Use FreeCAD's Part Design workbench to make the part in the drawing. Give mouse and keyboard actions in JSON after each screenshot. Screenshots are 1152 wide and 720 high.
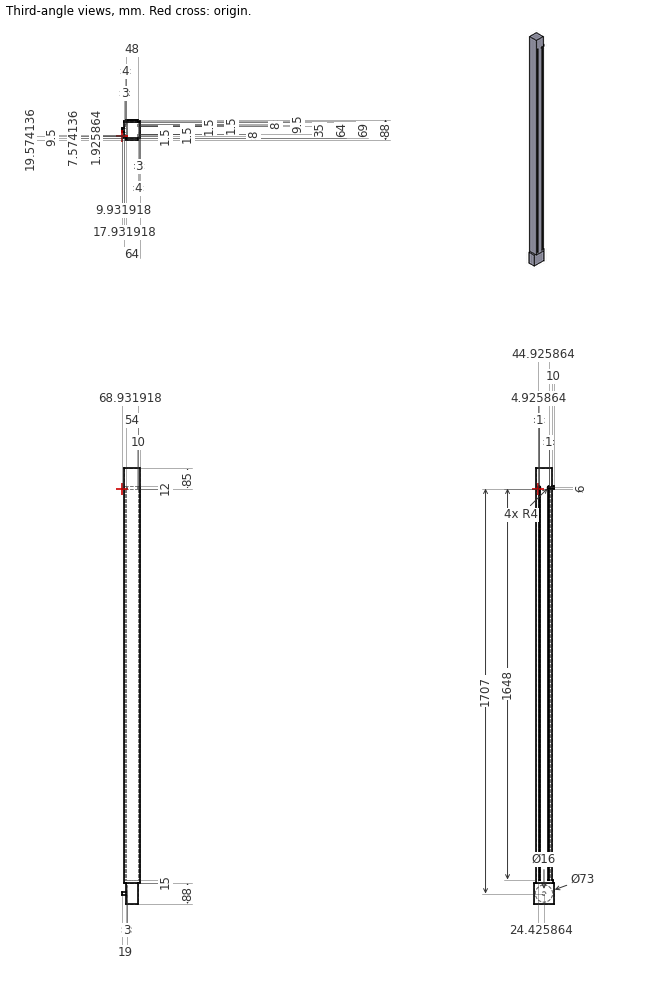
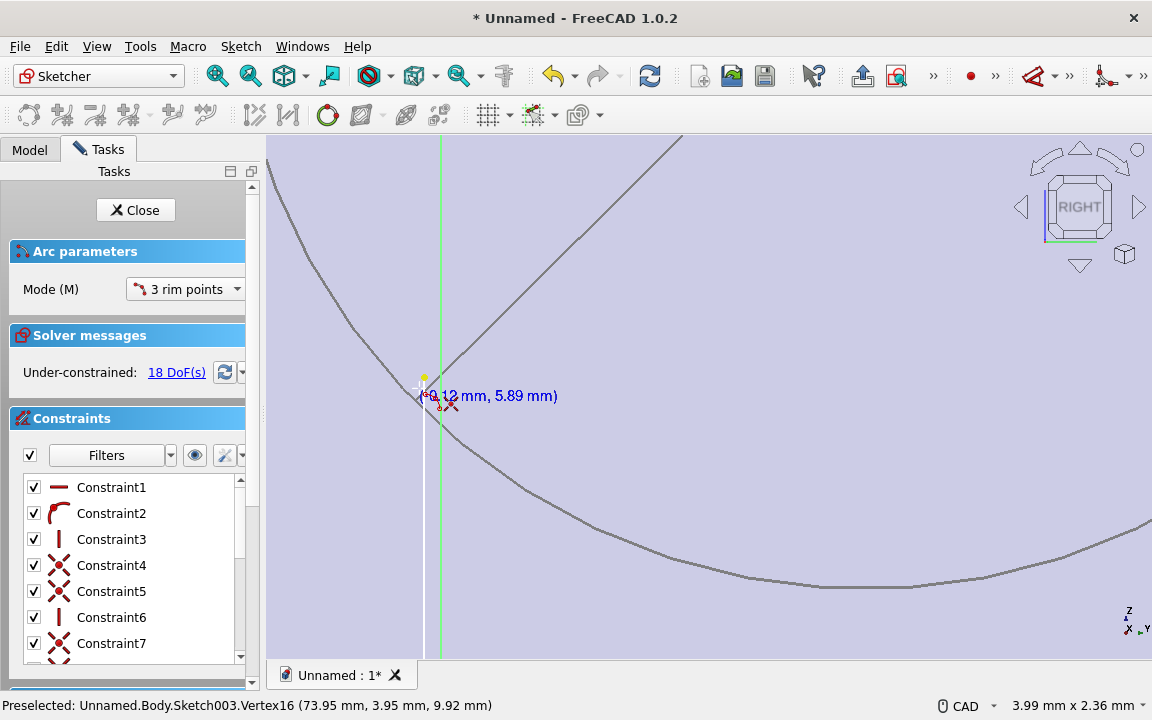
{"action": "left_click", "coordinate": [424, 377]}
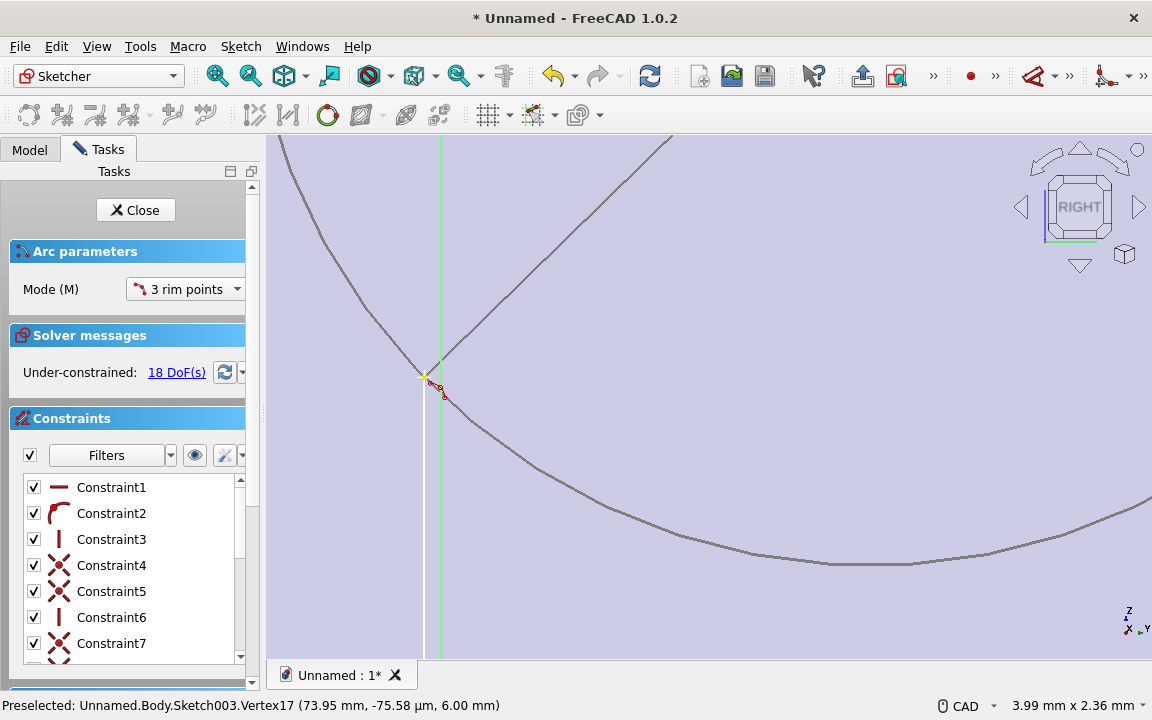
{"action": "scroll", "coordinate": [367, 386], "scroll_direction": "down", "scroll_amount": 15}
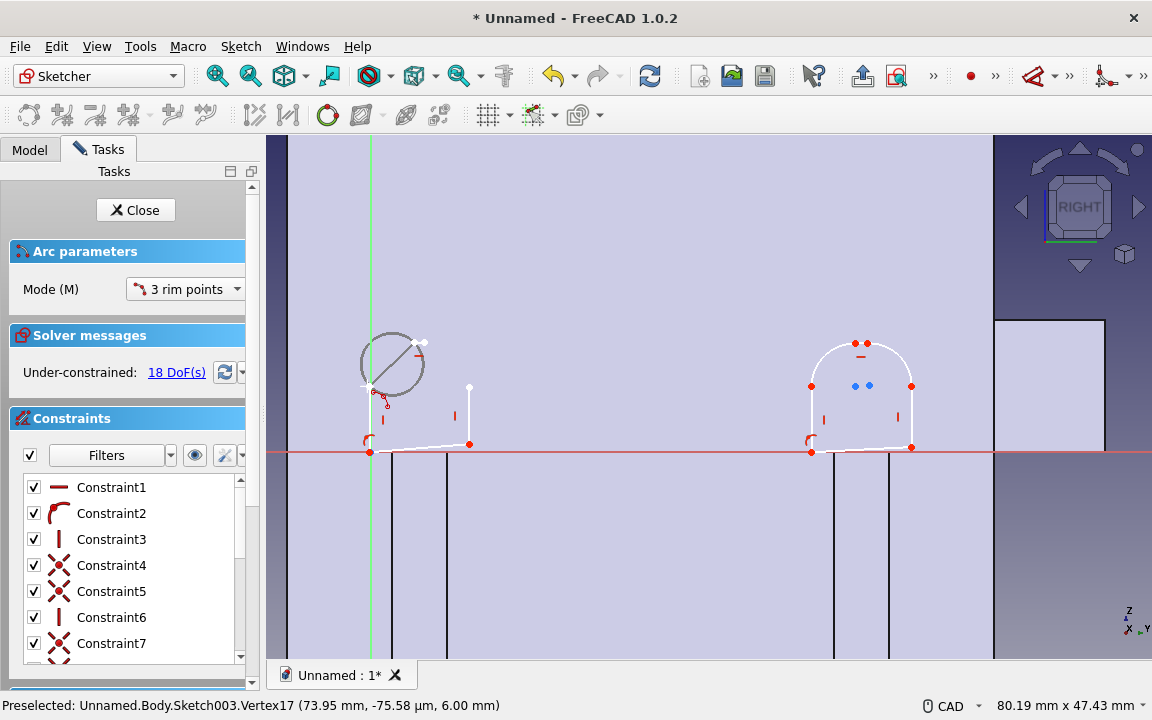
{"action": "scroll", "coordinate": [388, 350], "scroll_direction": "up", "scroll_amount": 2}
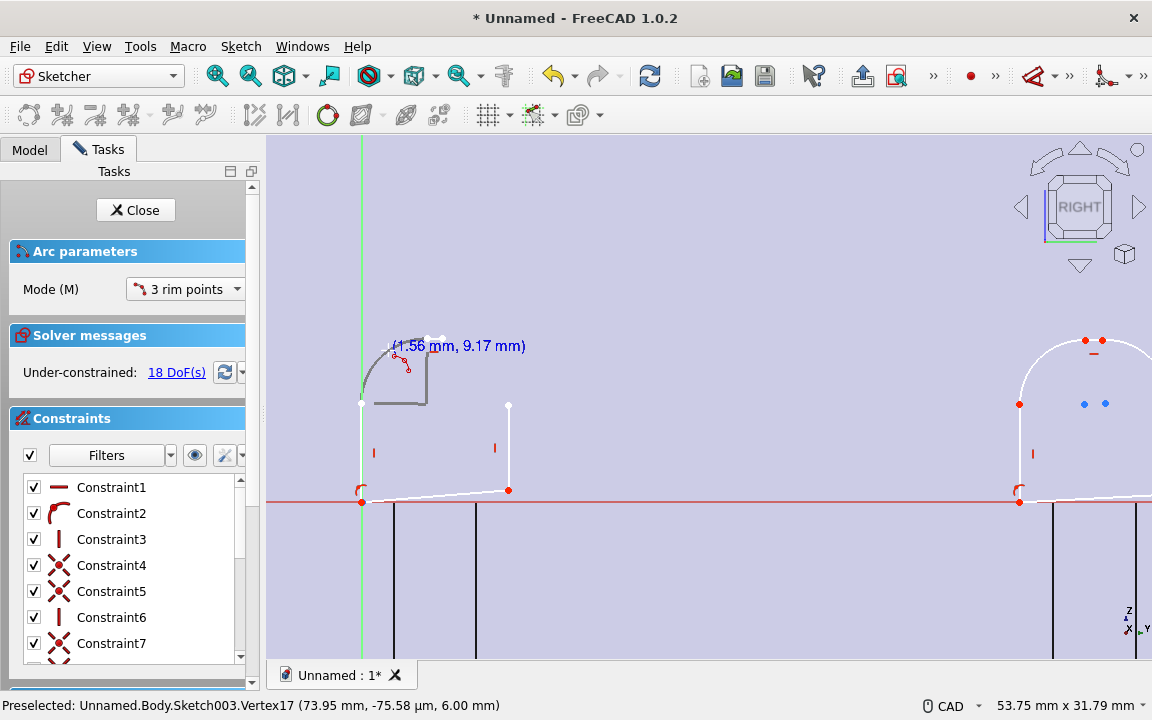
{"action": "left_click", "coordinate": [388, 350]}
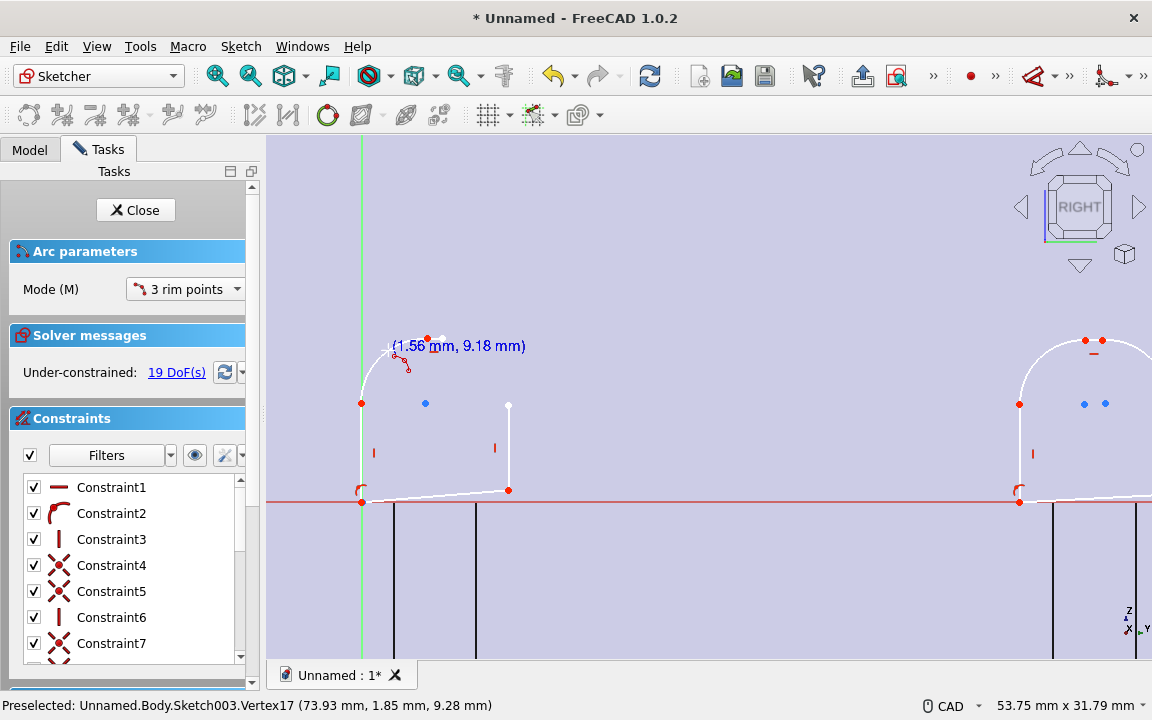
{"action": "left_click", "coordinate": [509, 405]}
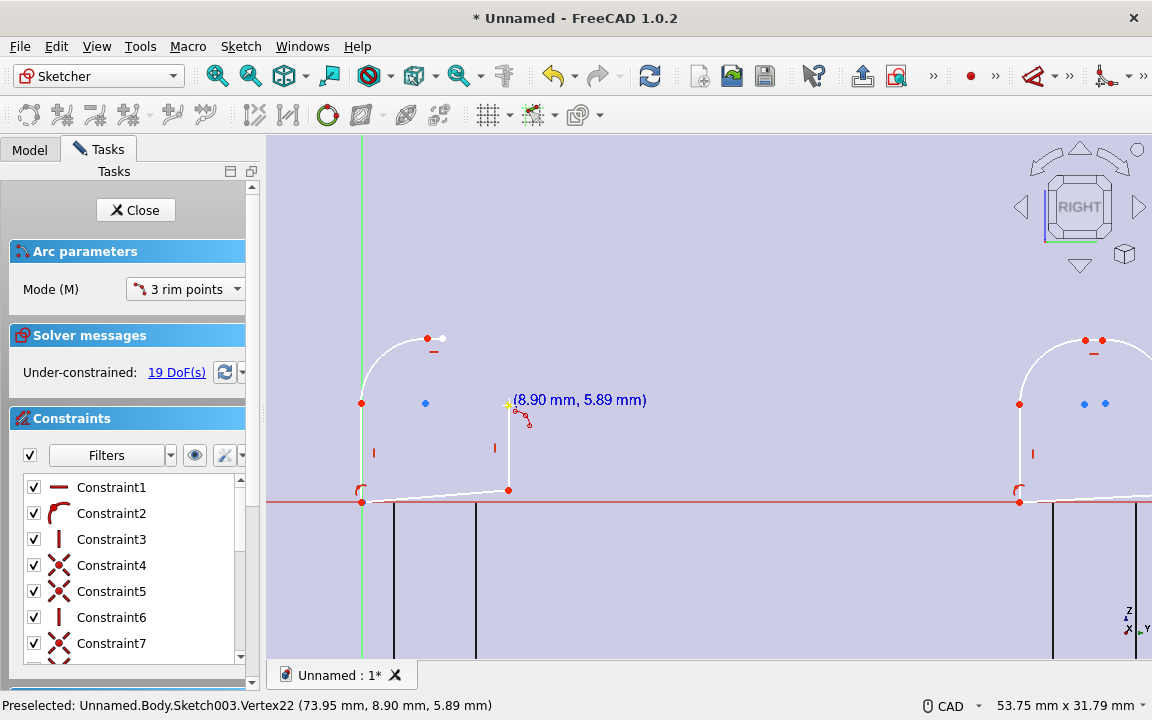
{"action": "scroll", "coordinate": [443, 338], "scroll_direction": "up", "scroll_amount": 4}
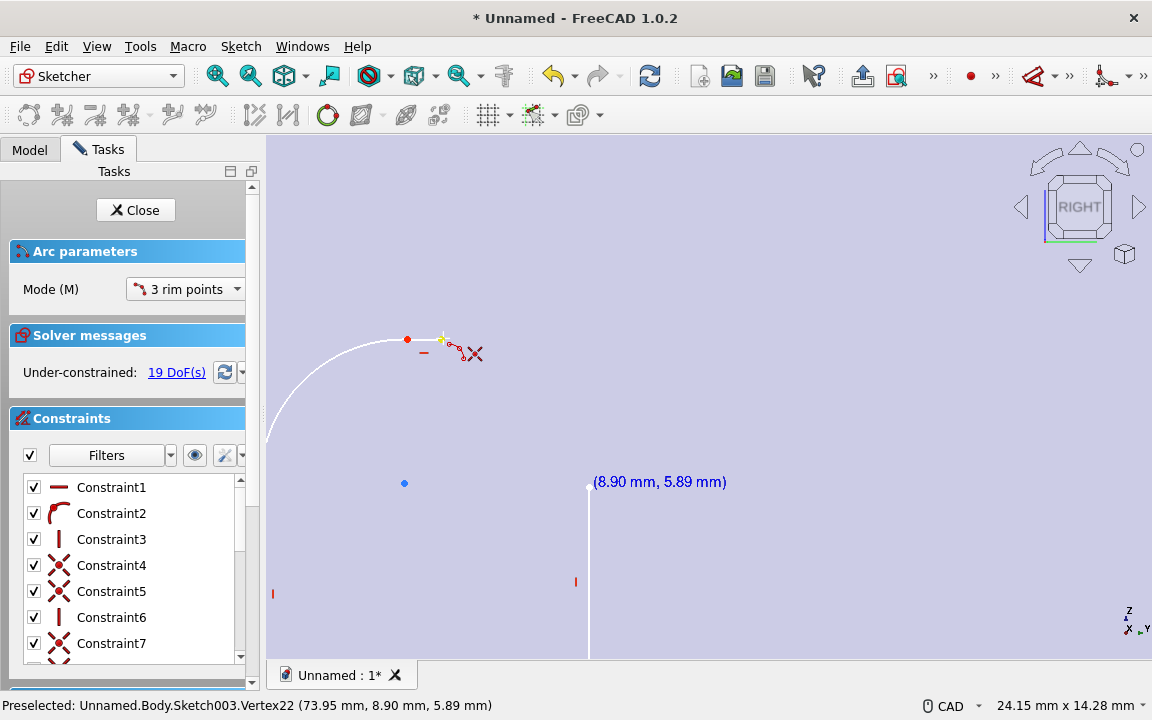
{"action": "left_click", "coordinate": [442, 340]}
{"action": "left_click", "coordinate": [547, 379]}
{"action": "key", "text": "Escape"}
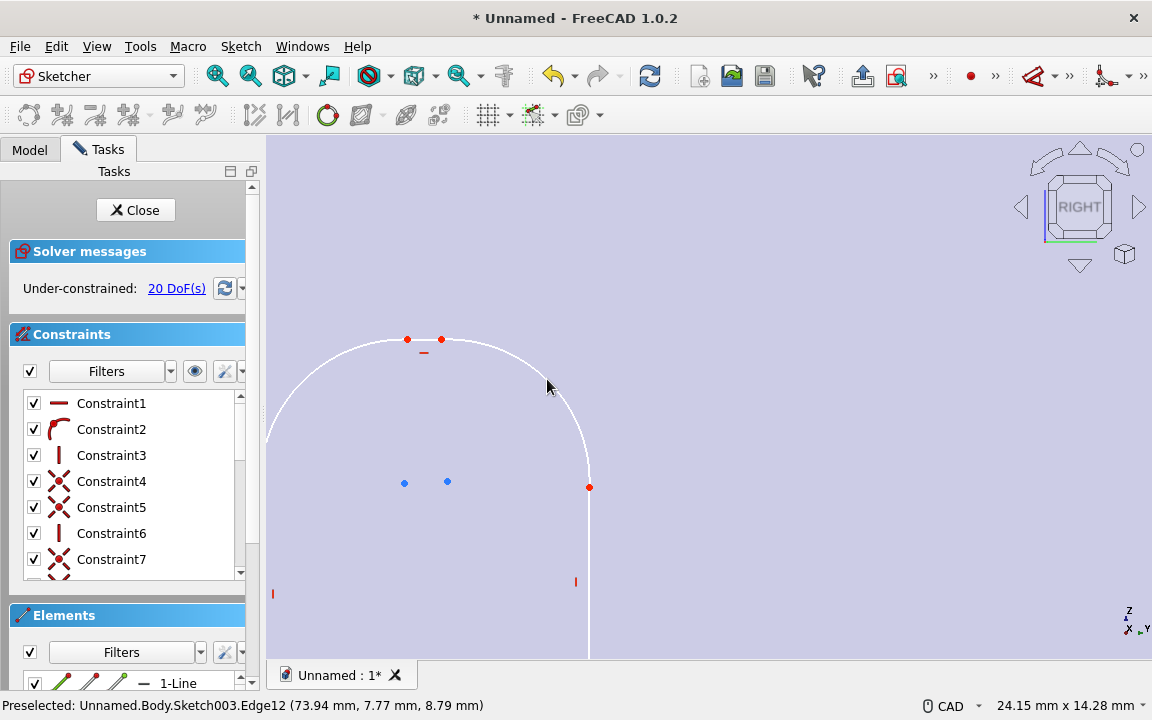
{"action": "scroll", "coordinate": [471, 357], "scroll_direction": "down", "scroll_amount": 7}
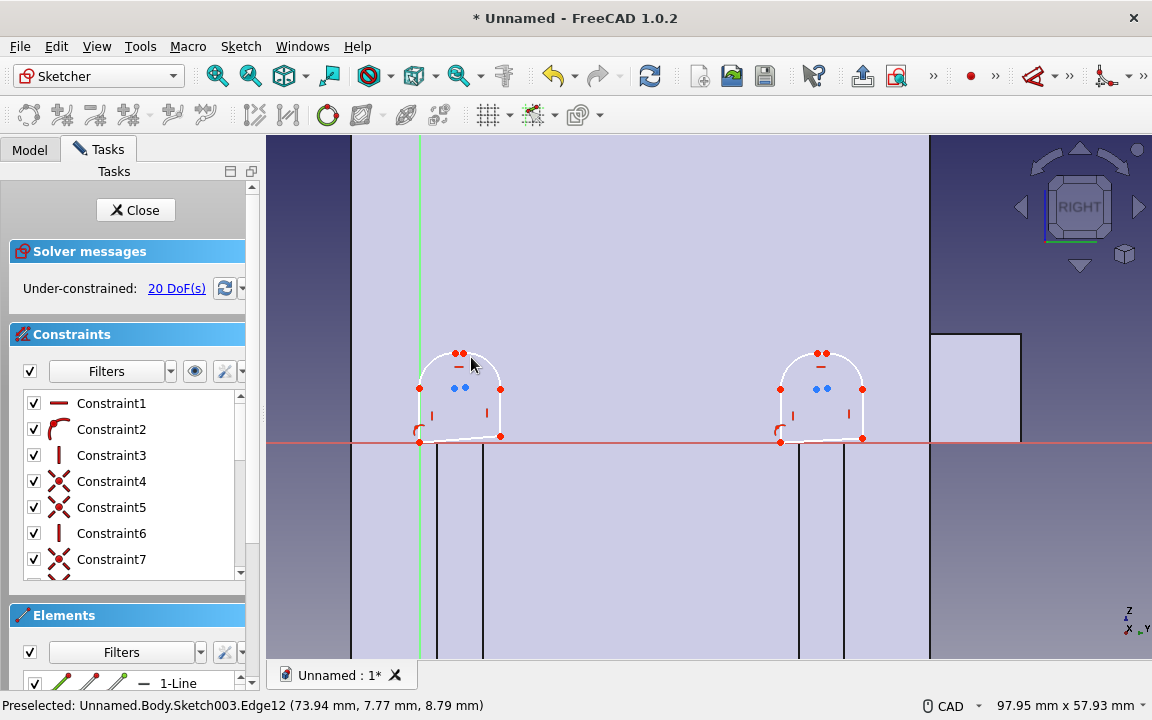
{"action": "scroll", "coordinate": [824, 354], "scroll_direction": "up", "scroll_amount": 9}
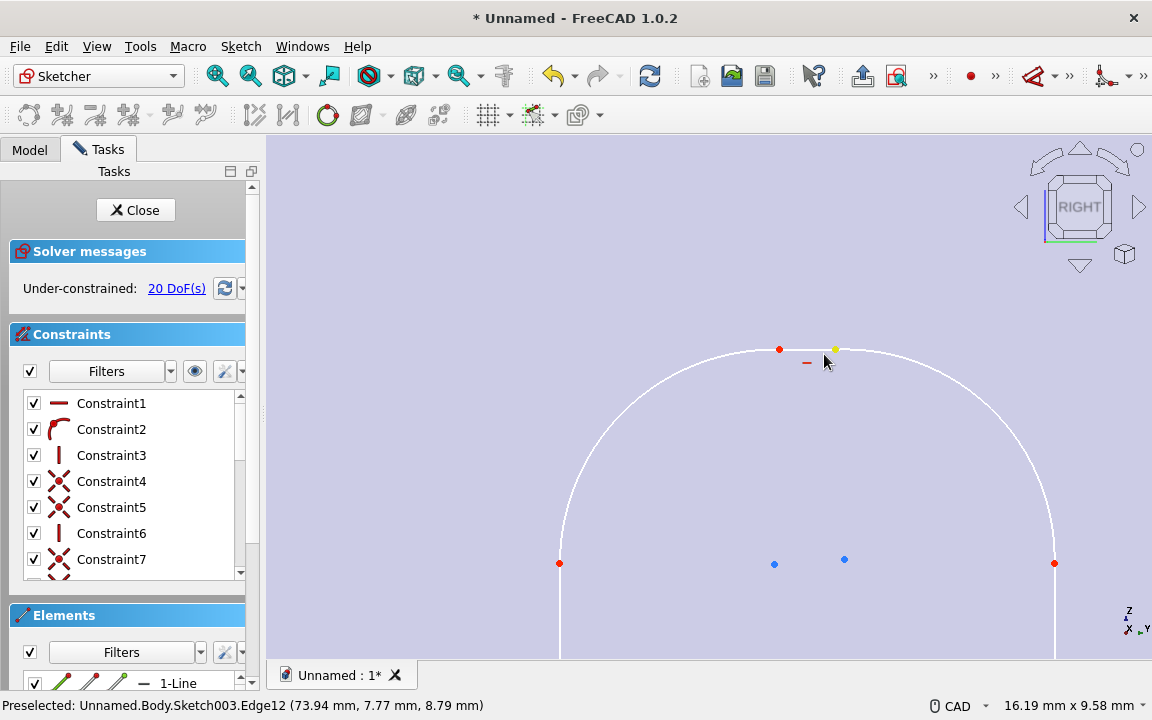
{"action": "left_click", "coordinate": [818, 350]}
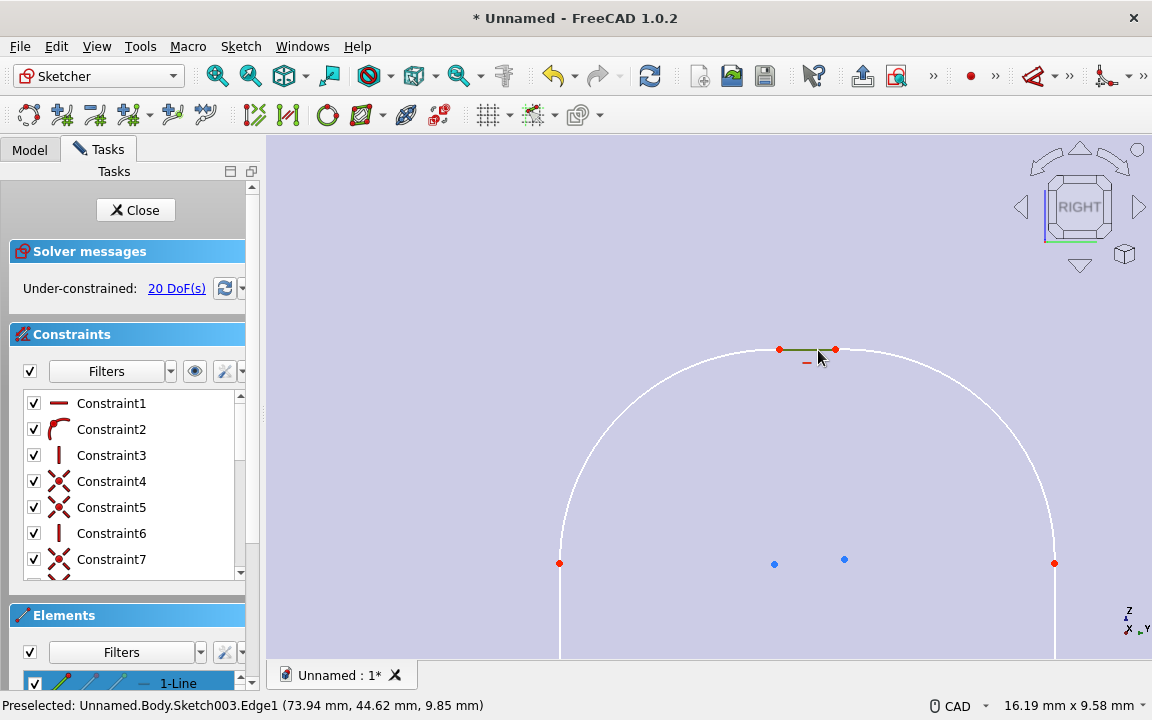
{"action": "scroll", "coordinate": [824, 354], "scroll_direction": "down", "scroll_amount": 9}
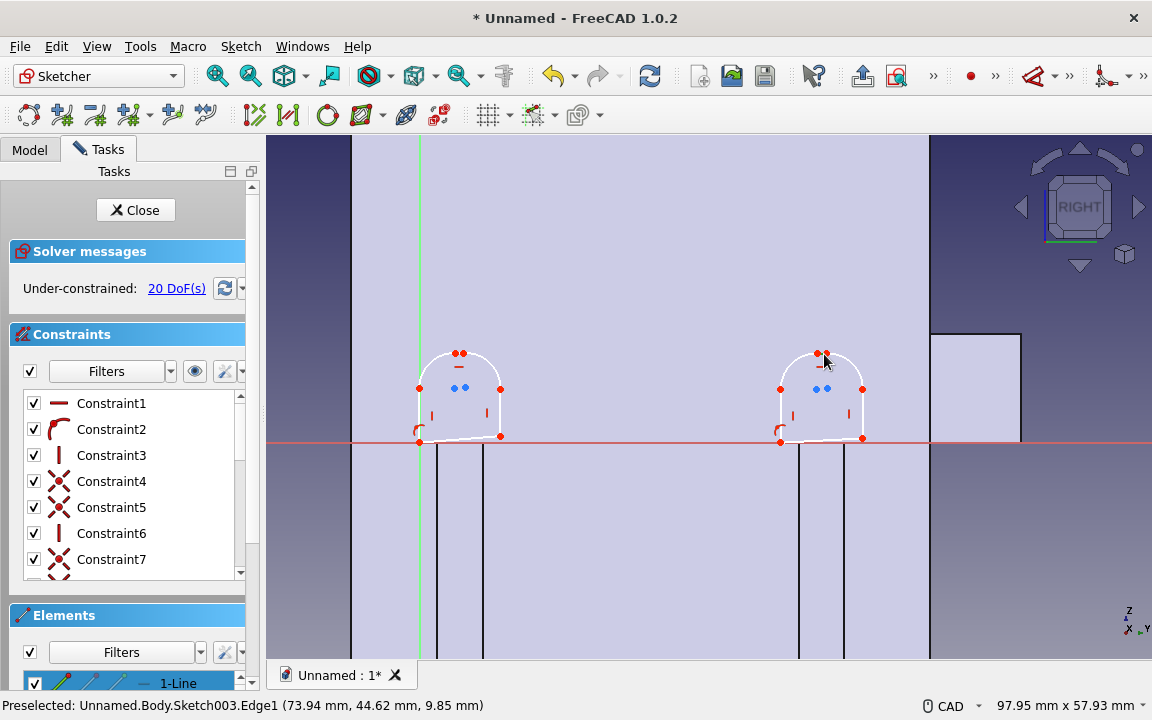
{"action": "left_click", "coordinate": [801, 357]}